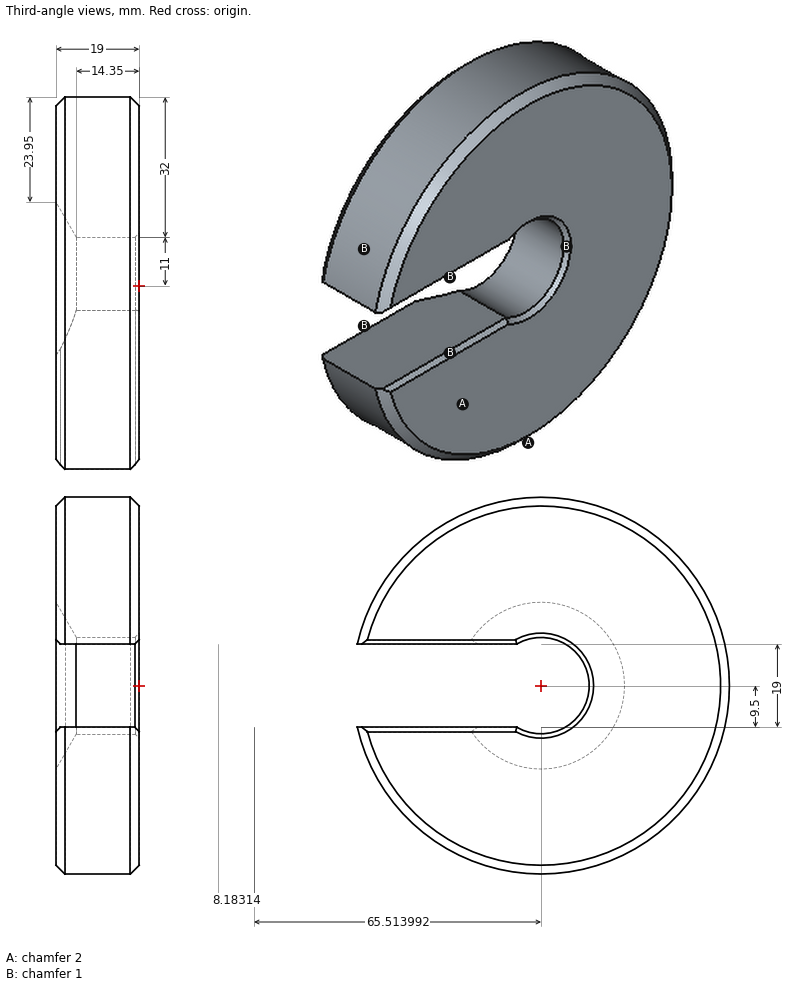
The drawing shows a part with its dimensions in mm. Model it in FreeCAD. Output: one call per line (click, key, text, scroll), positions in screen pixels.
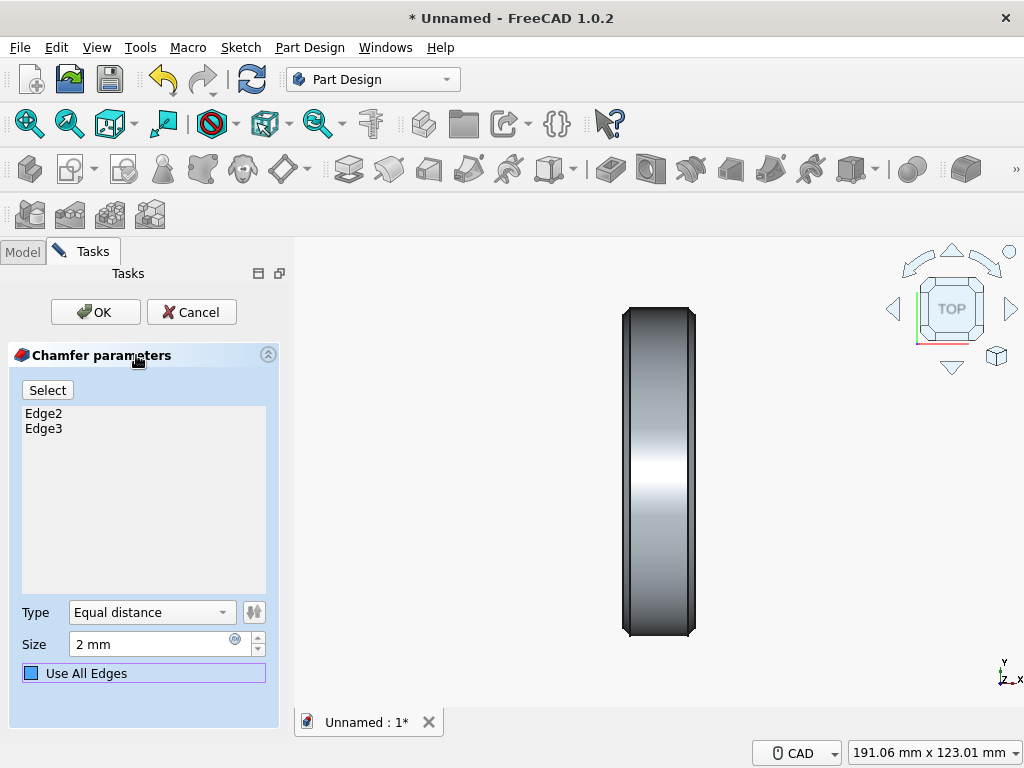
click(96, 312)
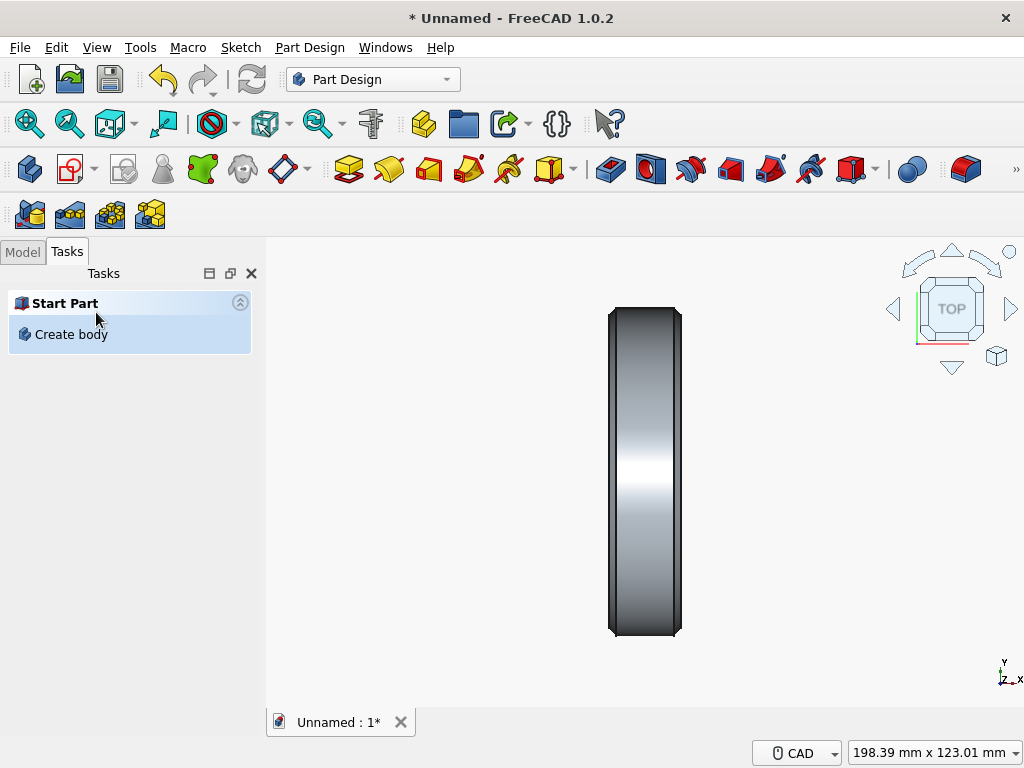
key(6)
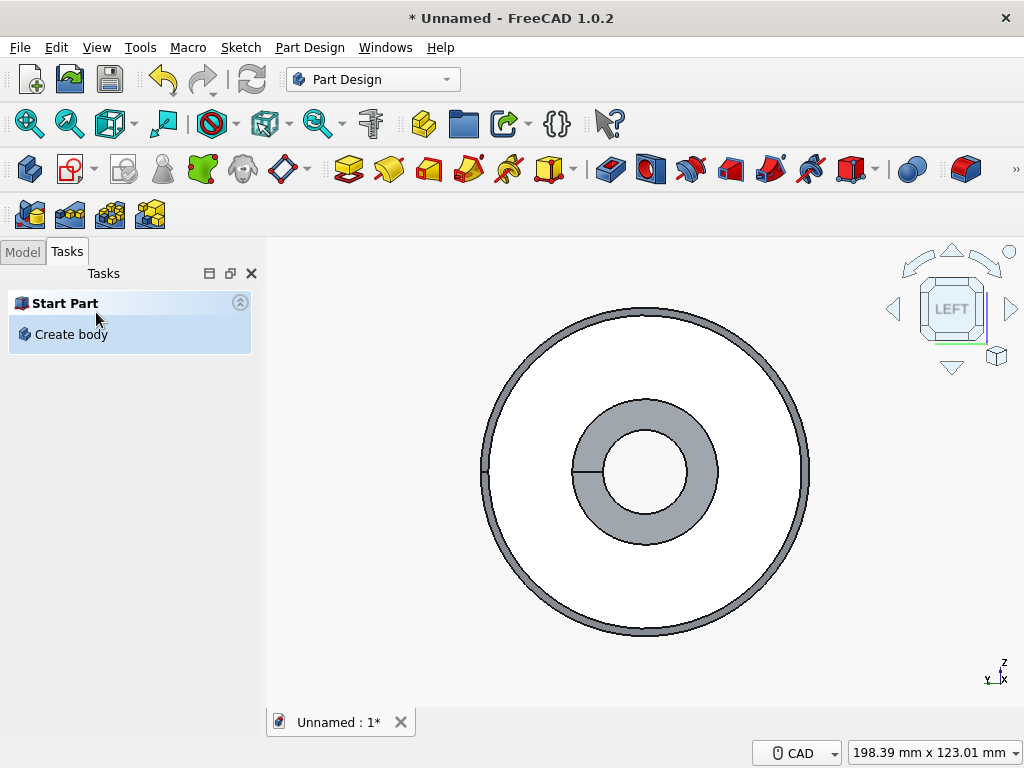
click(735, 561)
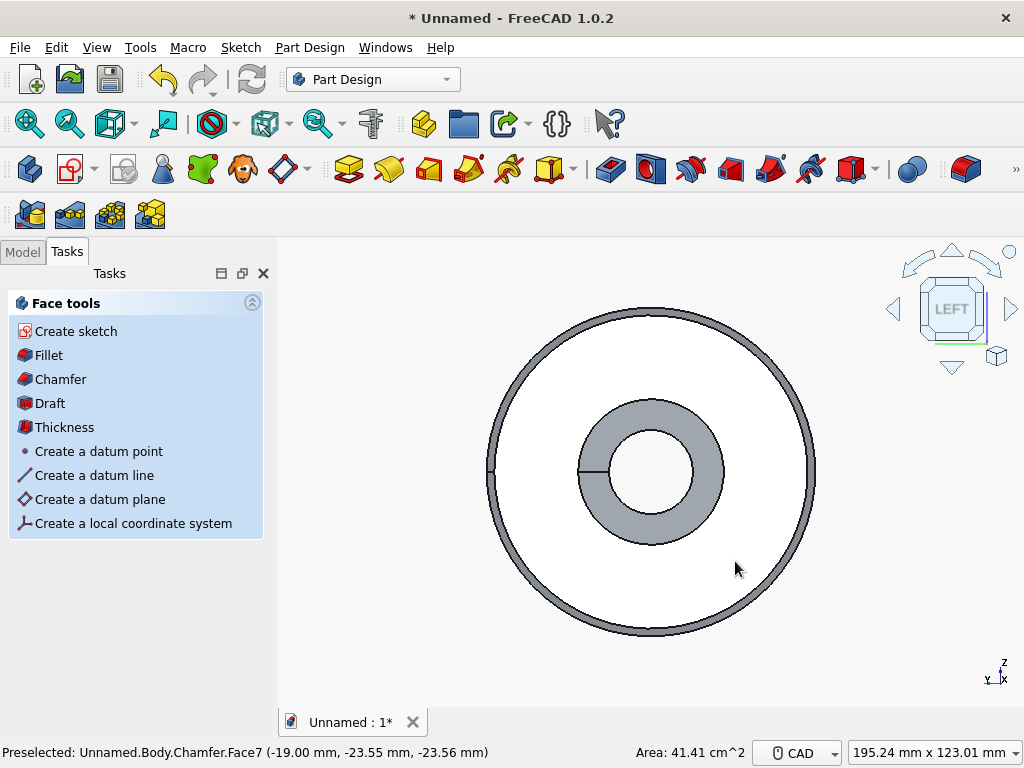
click(70, 170)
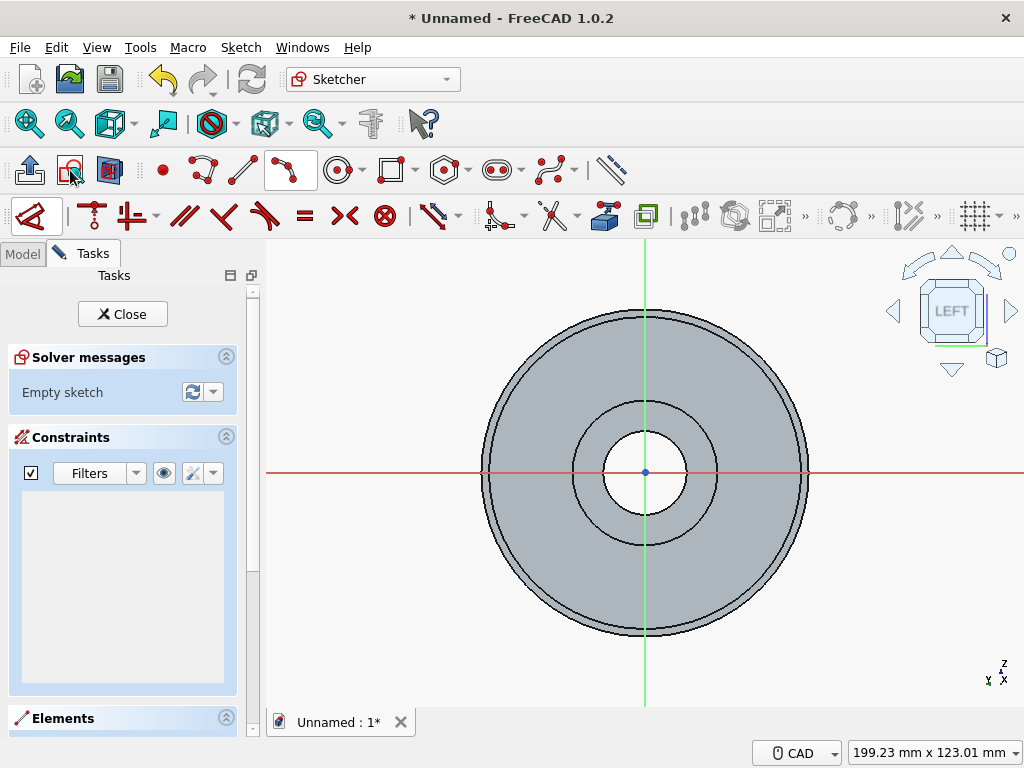
scroll(294, 473, down, 1)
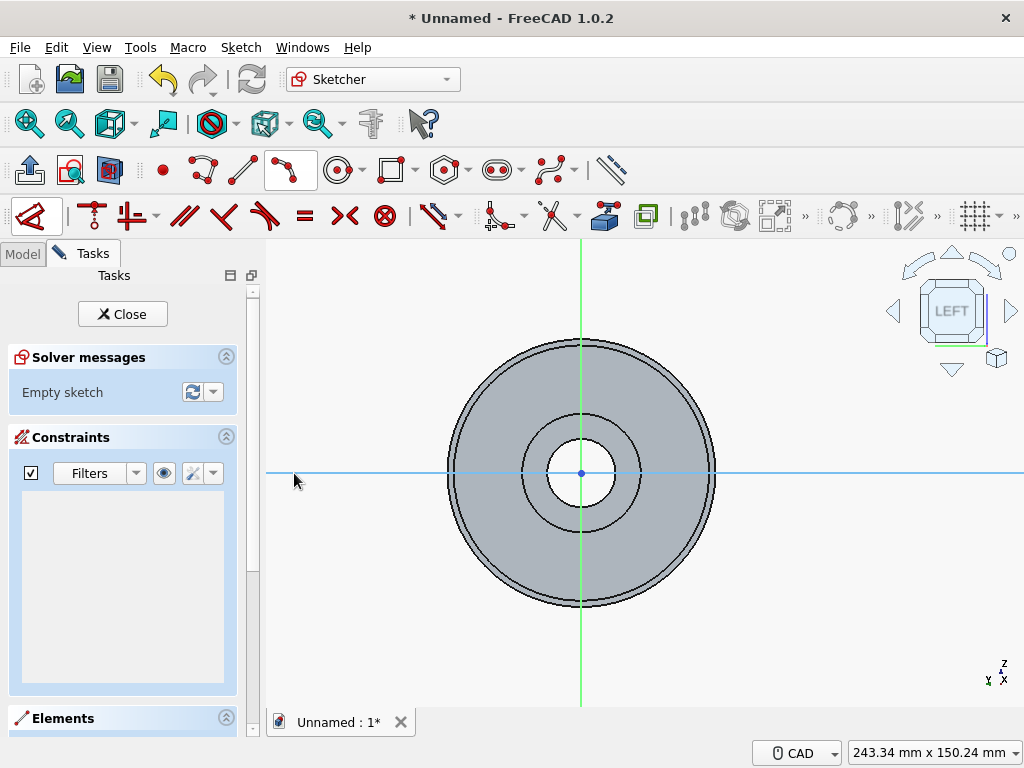
scroll(842, 473, up, 3)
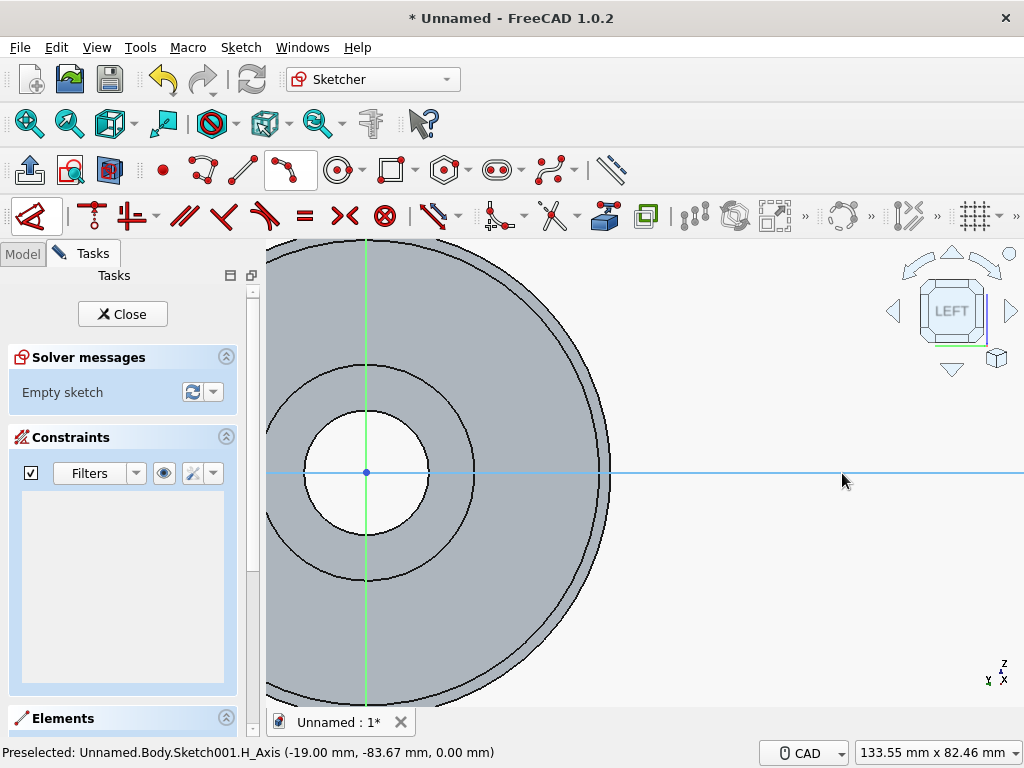
key(g)
key(m)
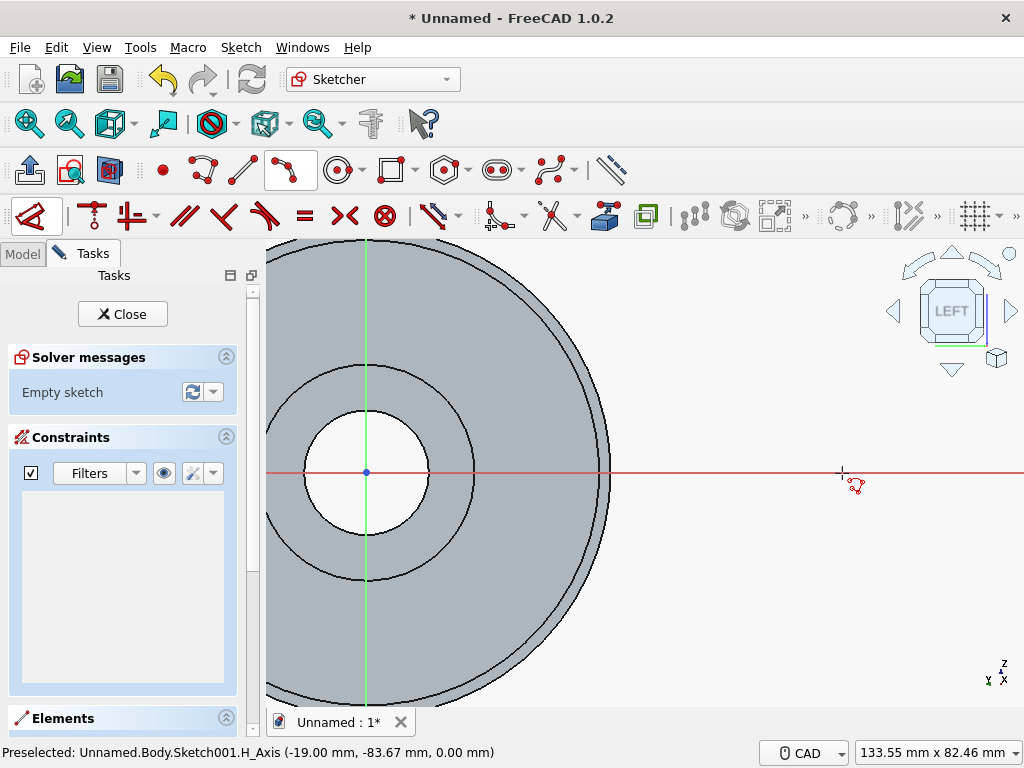
click(366, 527)
click(738, 527)
click(785, 419)
click(375, 419)
click(366, 528)
key(Escape)
key(Escape)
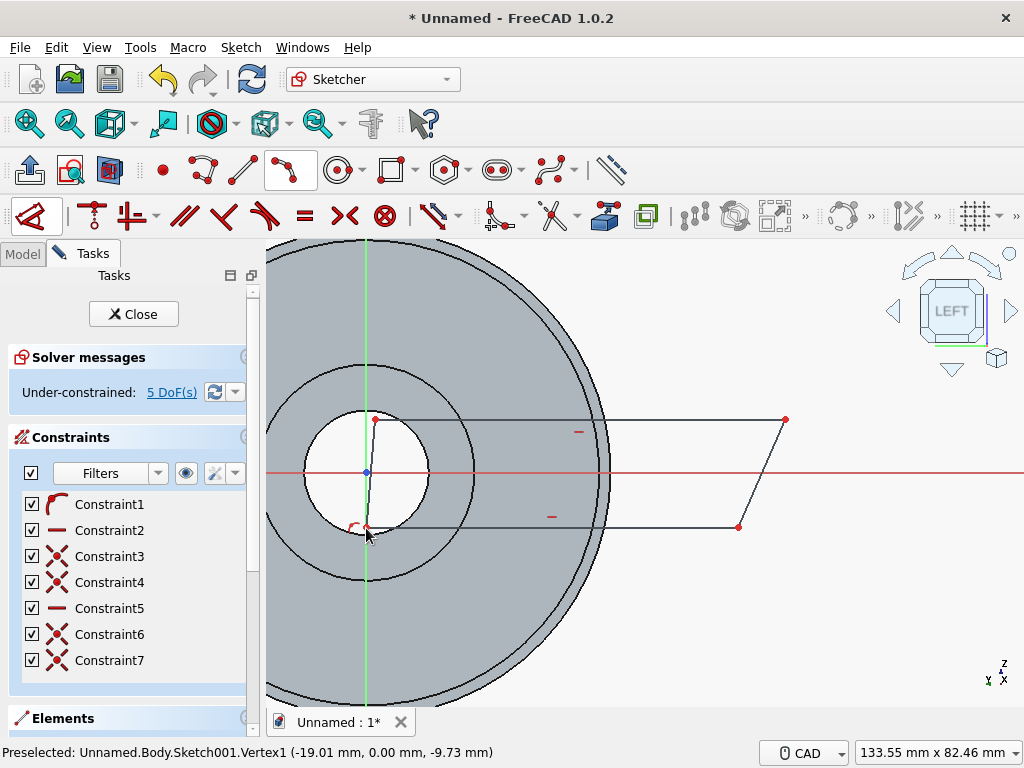
click(369, 496)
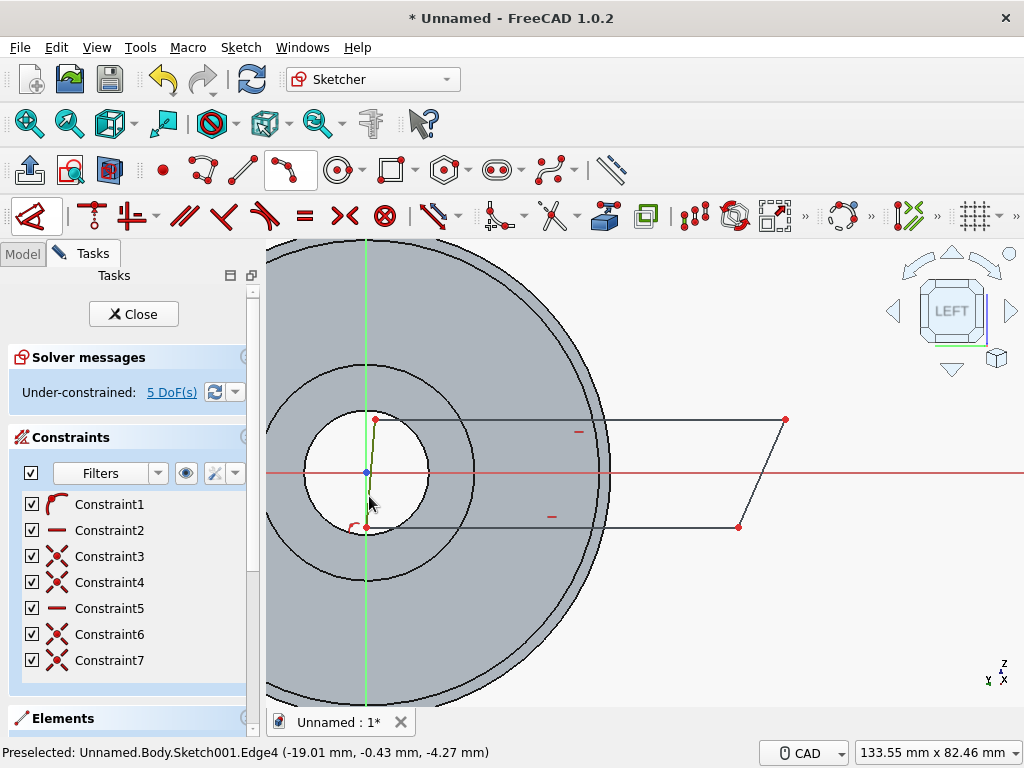
click(158, 216)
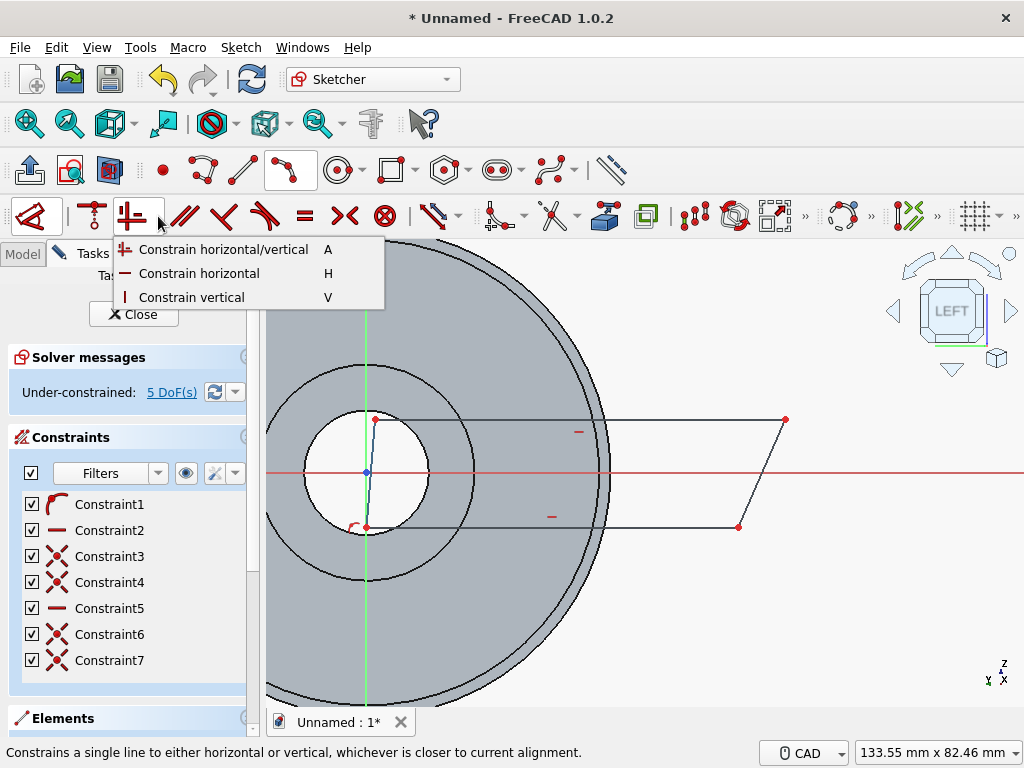
click(249, 297)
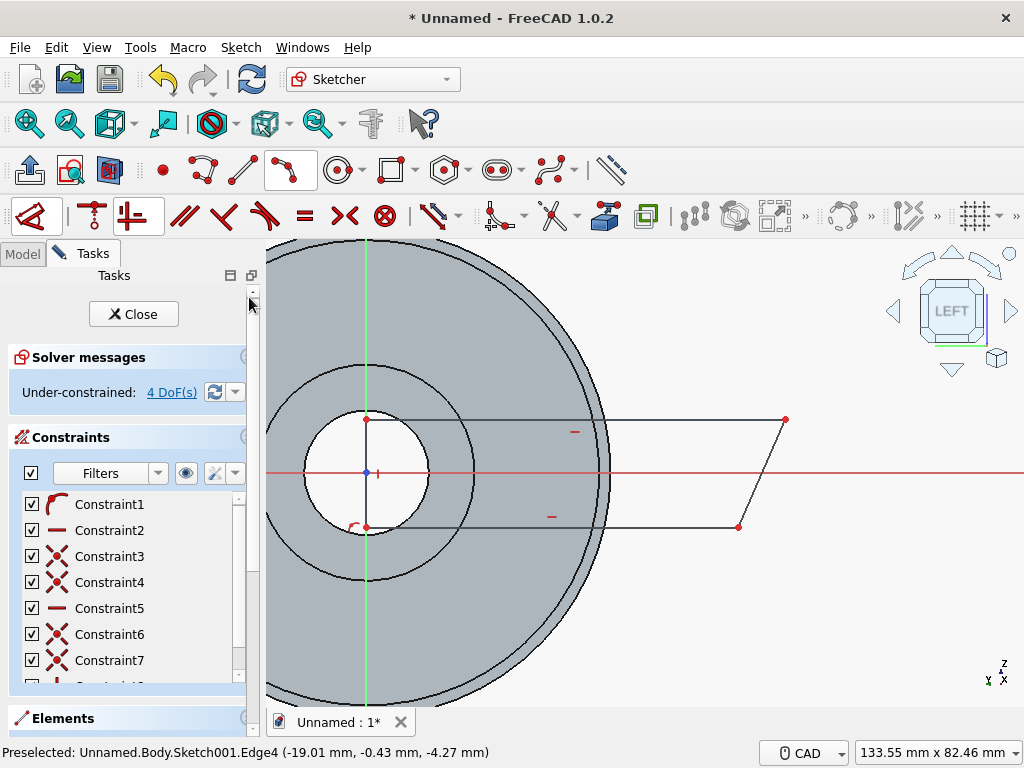
click(366, 452)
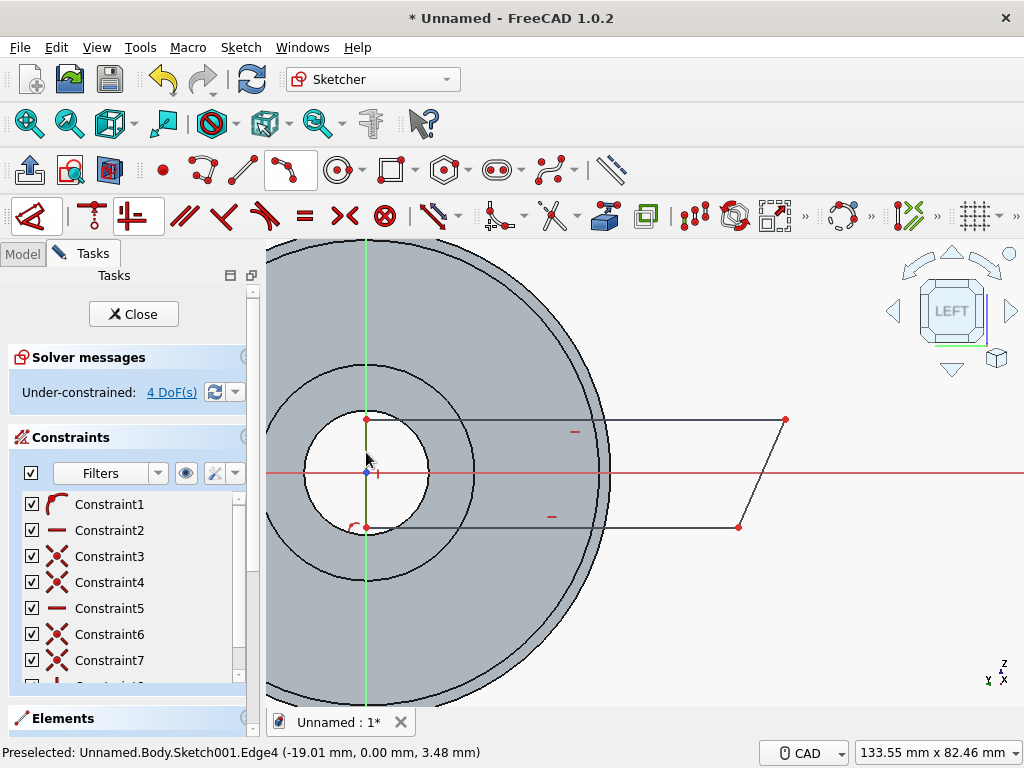
key(i)